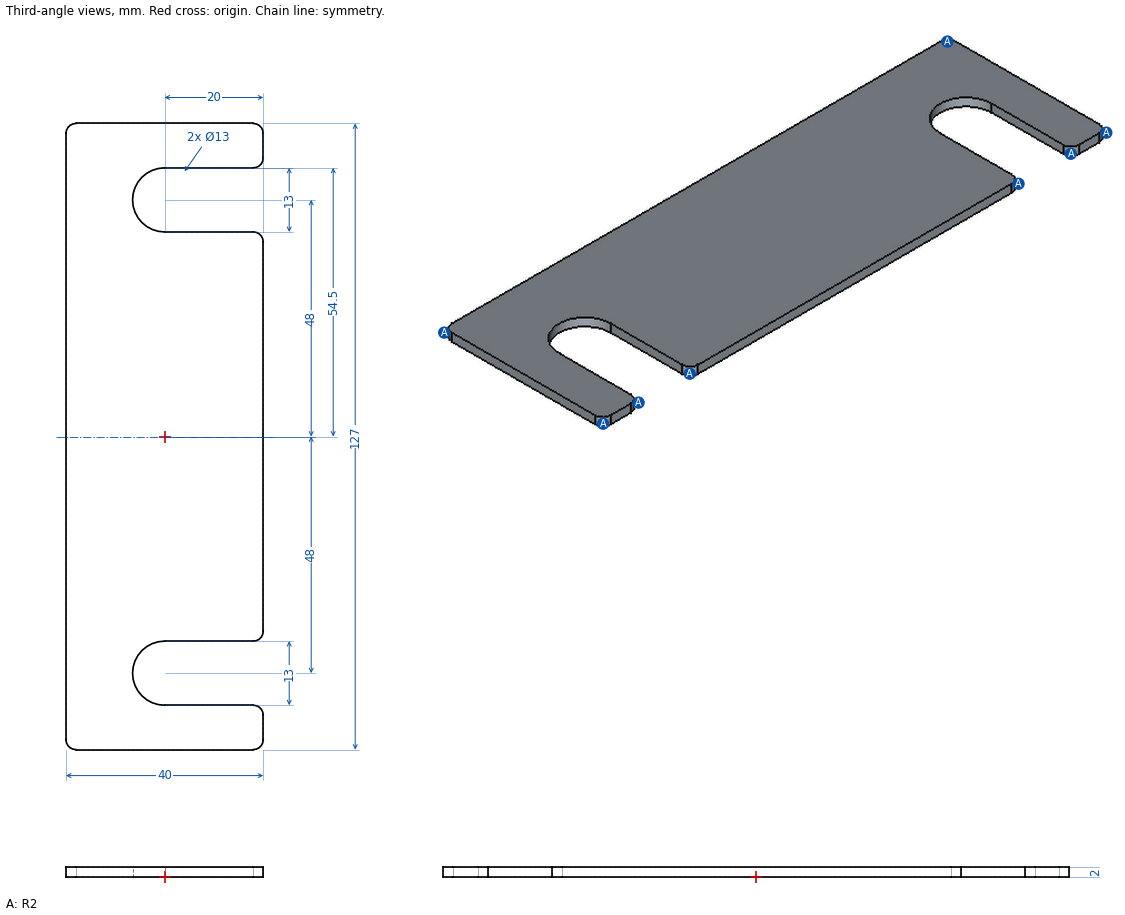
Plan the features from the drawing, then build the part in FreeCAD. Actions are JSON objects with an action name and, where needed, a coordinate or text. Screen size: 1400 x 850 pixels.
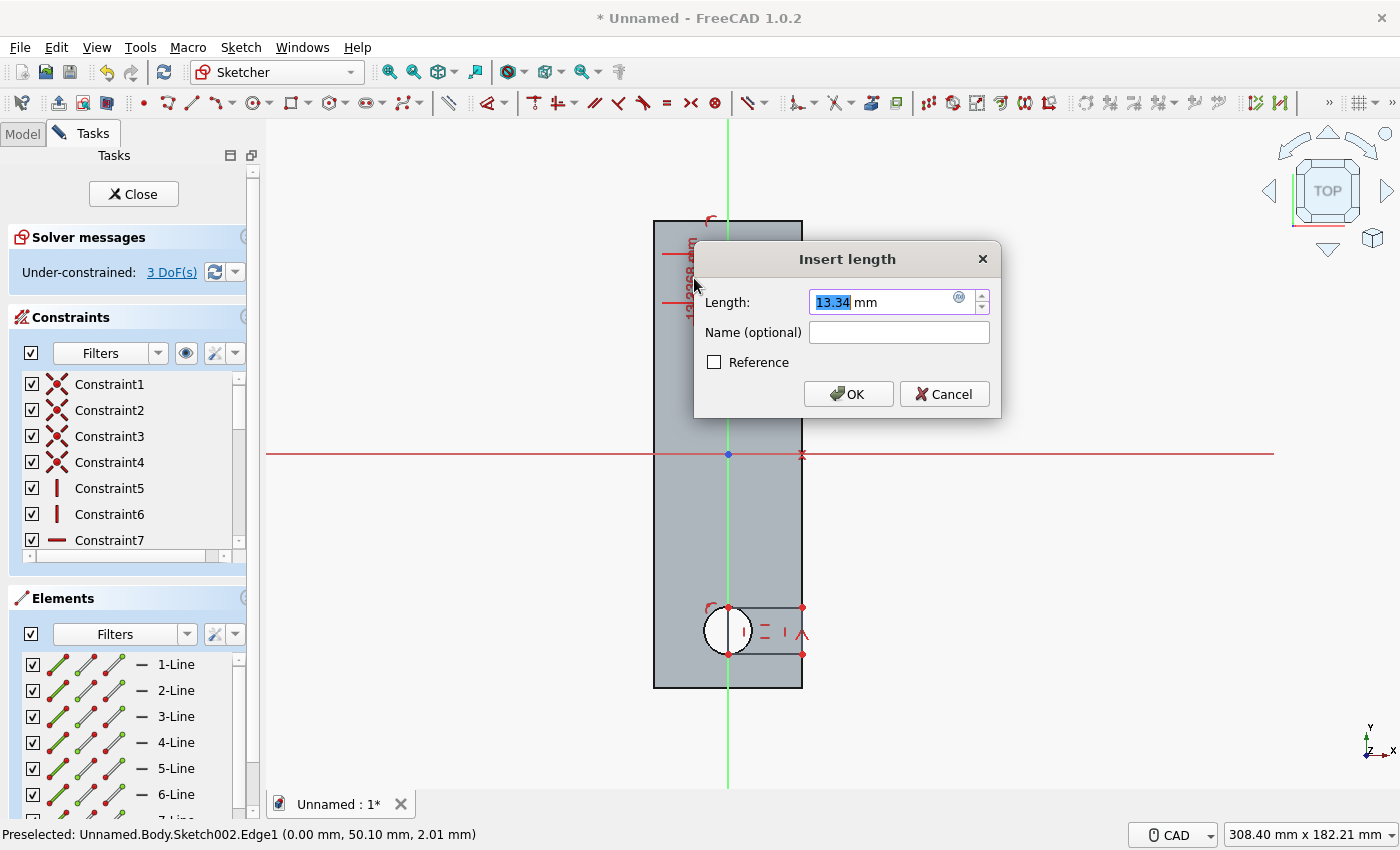
{"action": "type", "text": "13"}
{"action": "key", "text": "Return"}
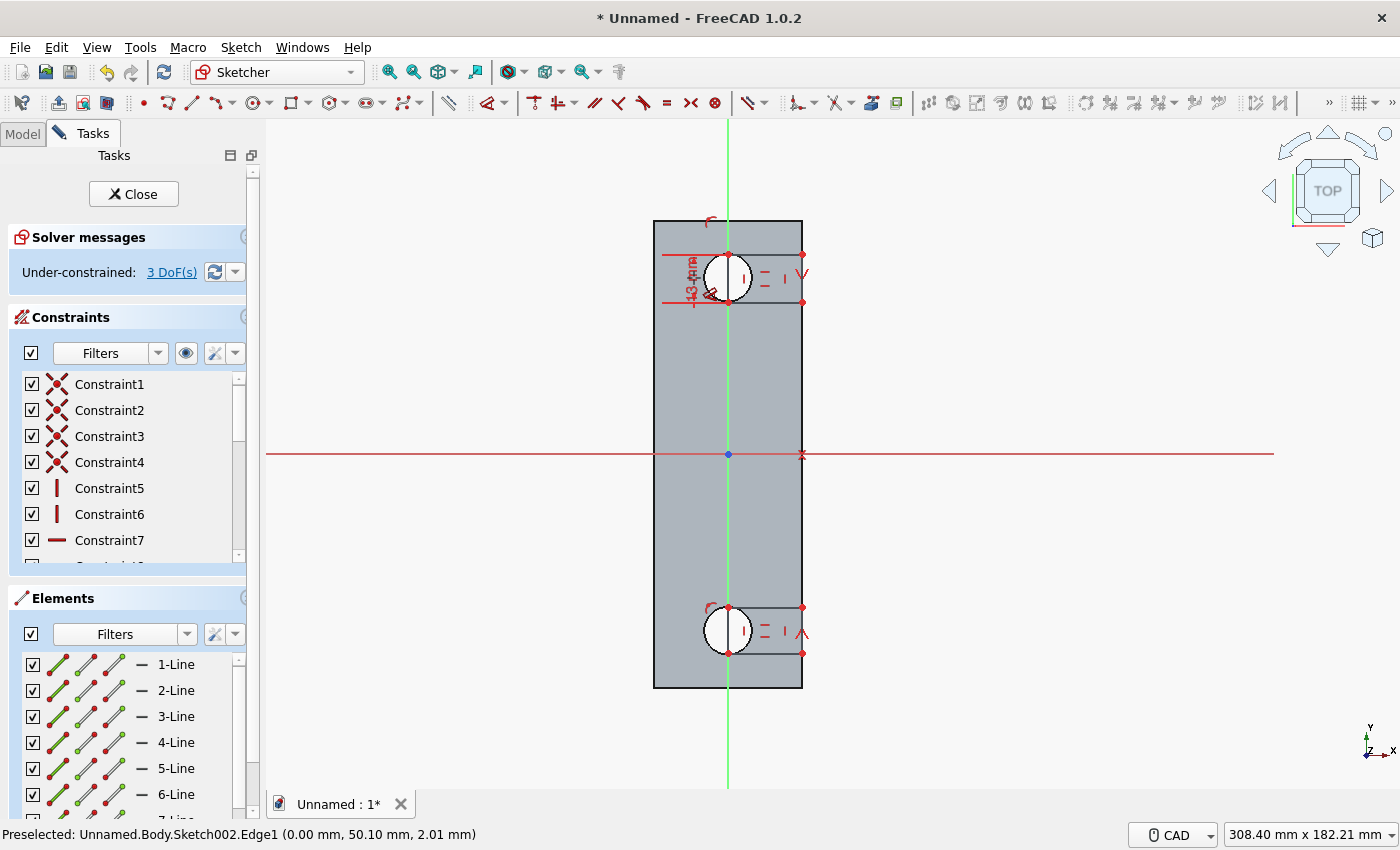
{"action": "left_click", "coordinate": [750, 303]}
{"action": "left_click", "coordinate": [765, 269]}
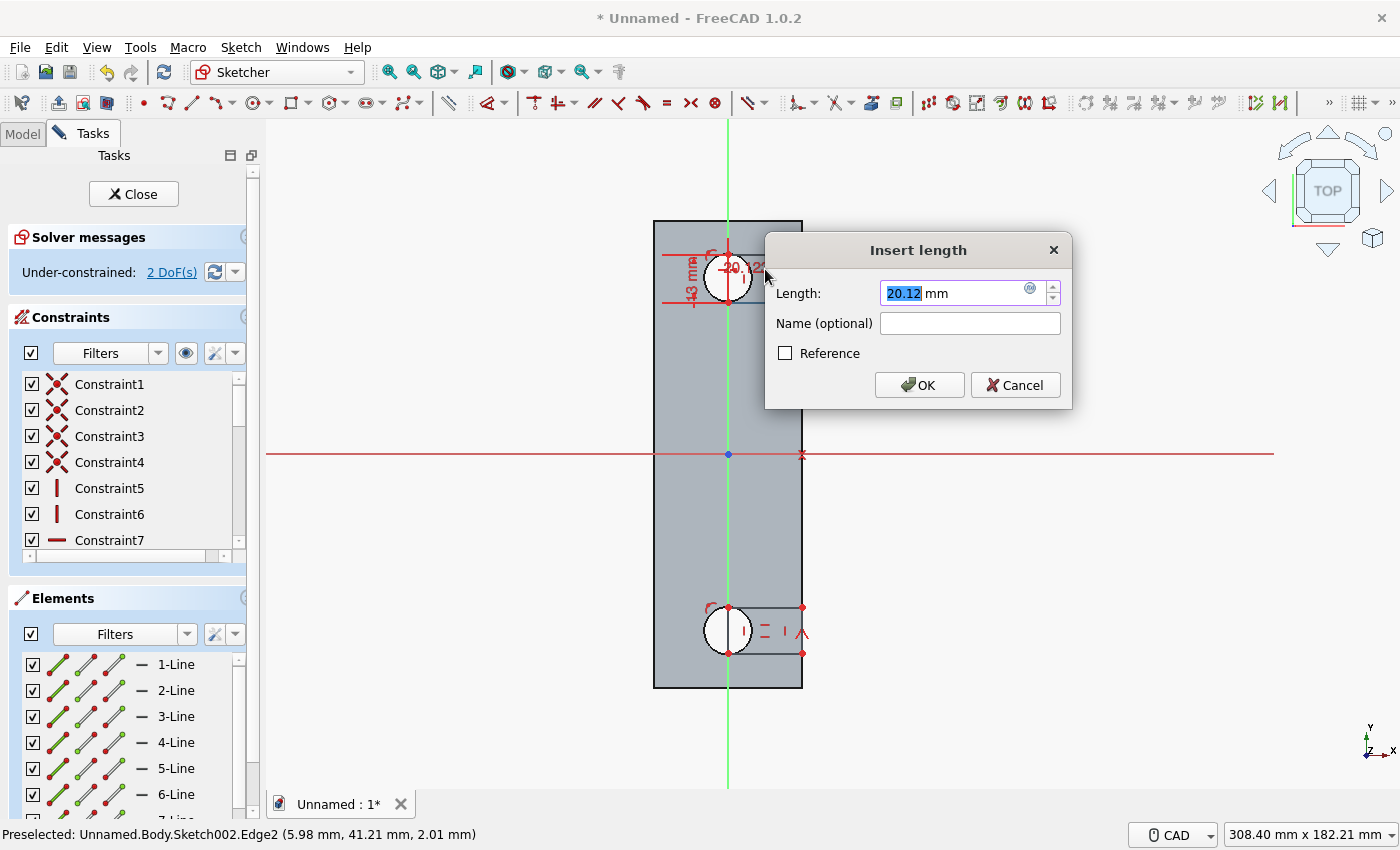
{"action": "type", "text": "20"}
{"action": "key", "text": "Return"}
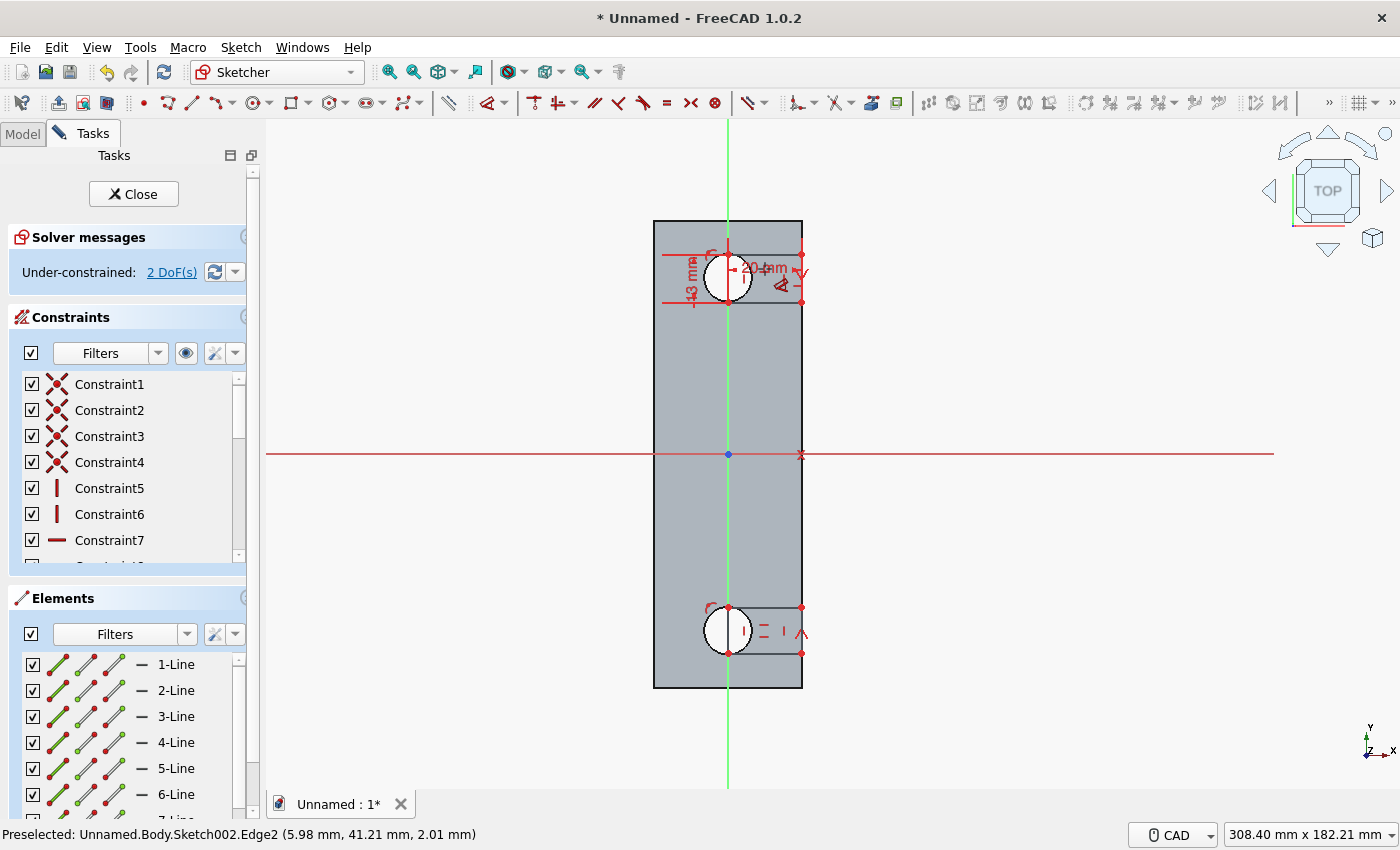
{"action": "left_click", "coordinate": [728, 622]}
{"action": "left_click", "coordinate": [694, 631]}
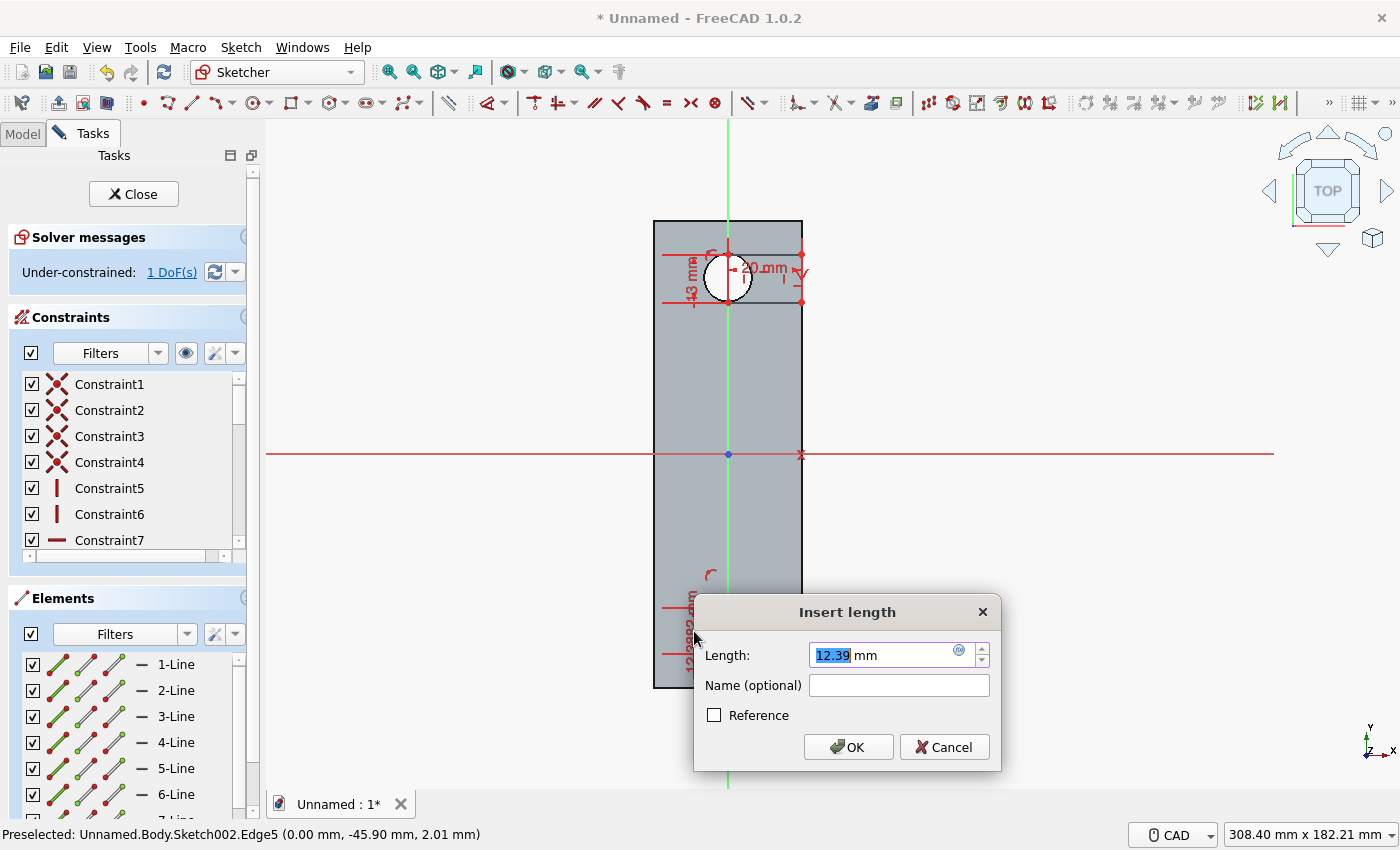
{"action": "type", "text": "13"}
{"action": "key", "text": "Return"}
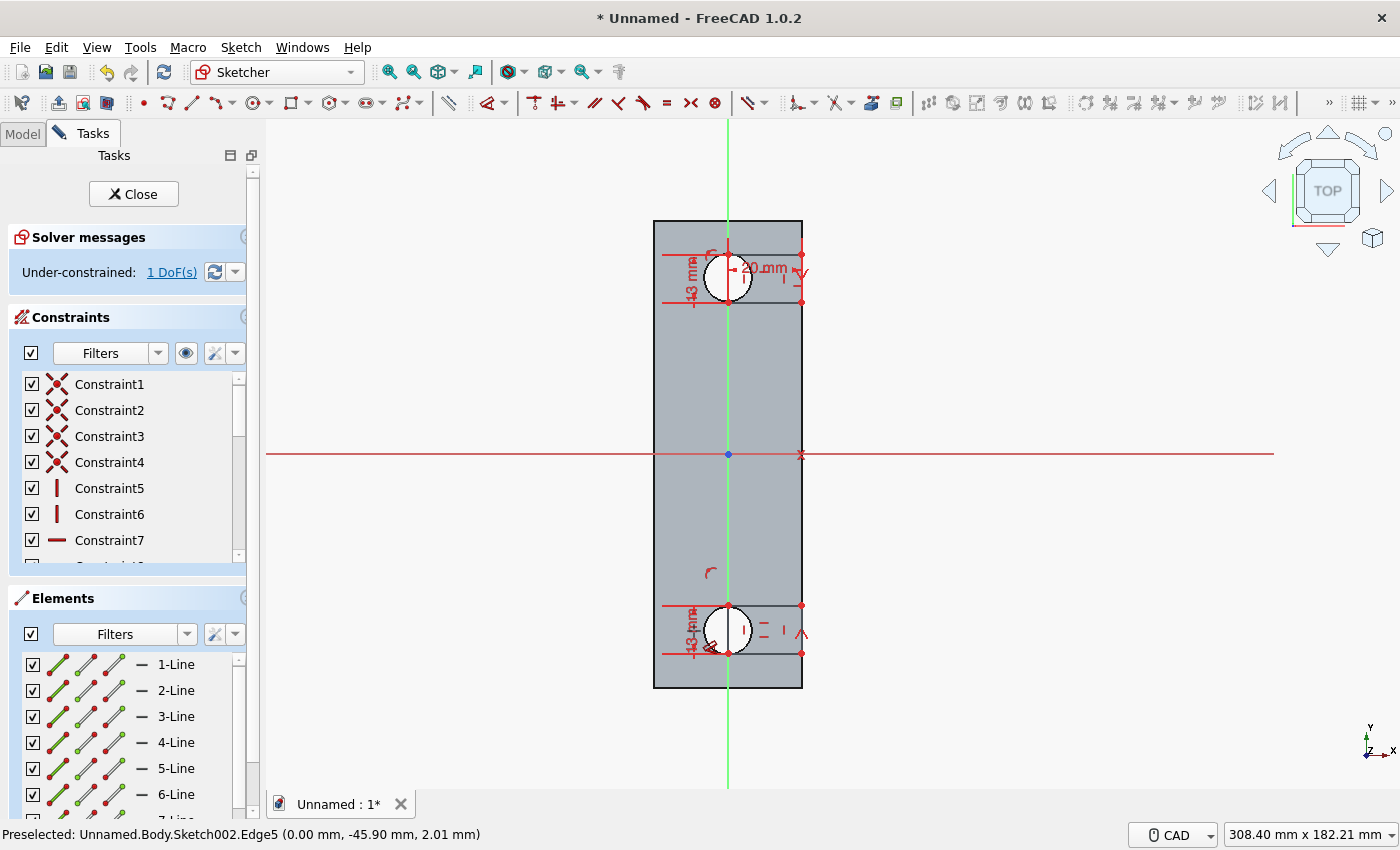
{"action": "left_click", "coordinate": [728, 255]}
{"action": "left_click", "coordinate": [694, 355]}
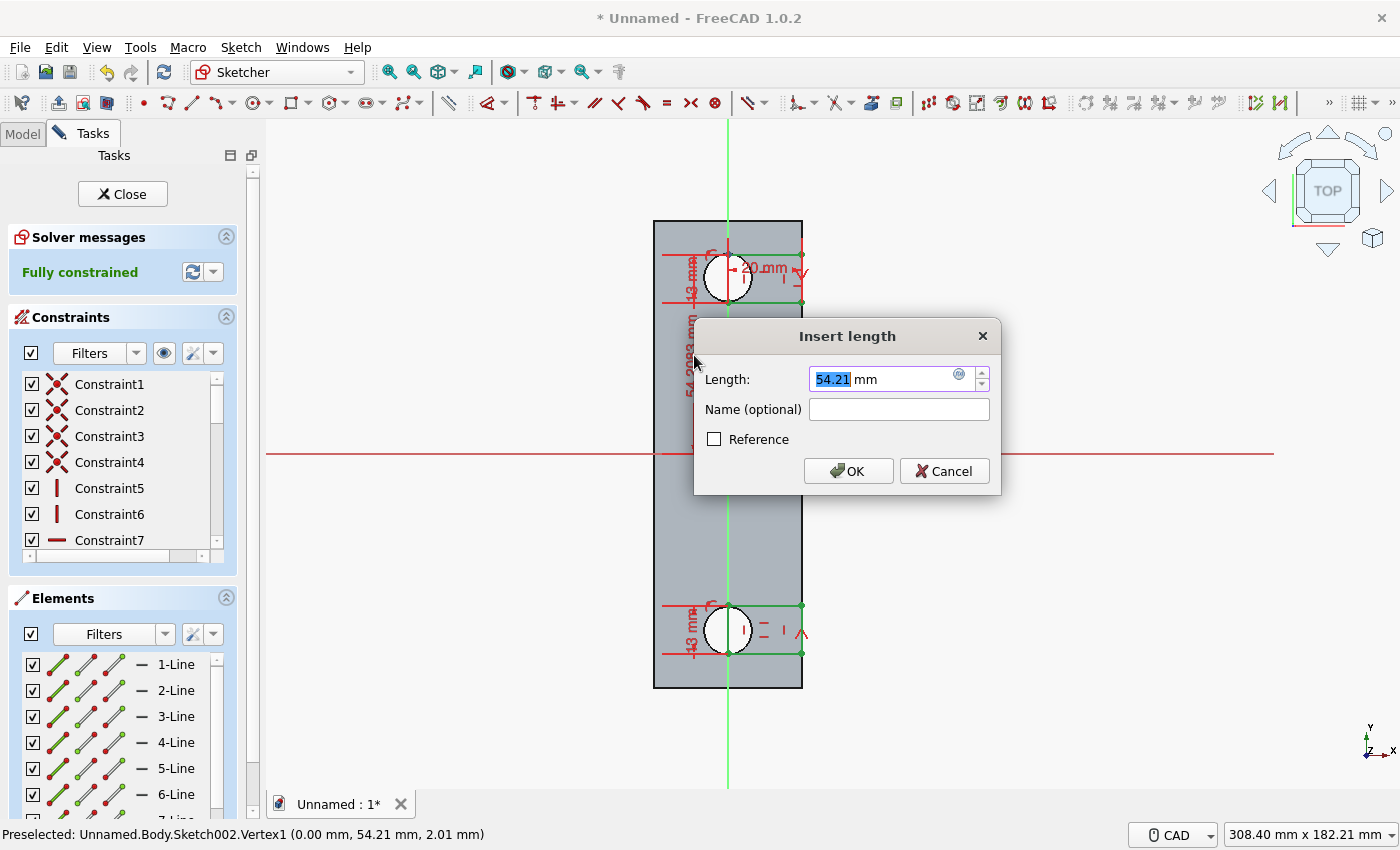
{"action": "type", "text": "54.5"}
{"action": "key", "text": "Return"}
{"action": "key", "text": "Escape"}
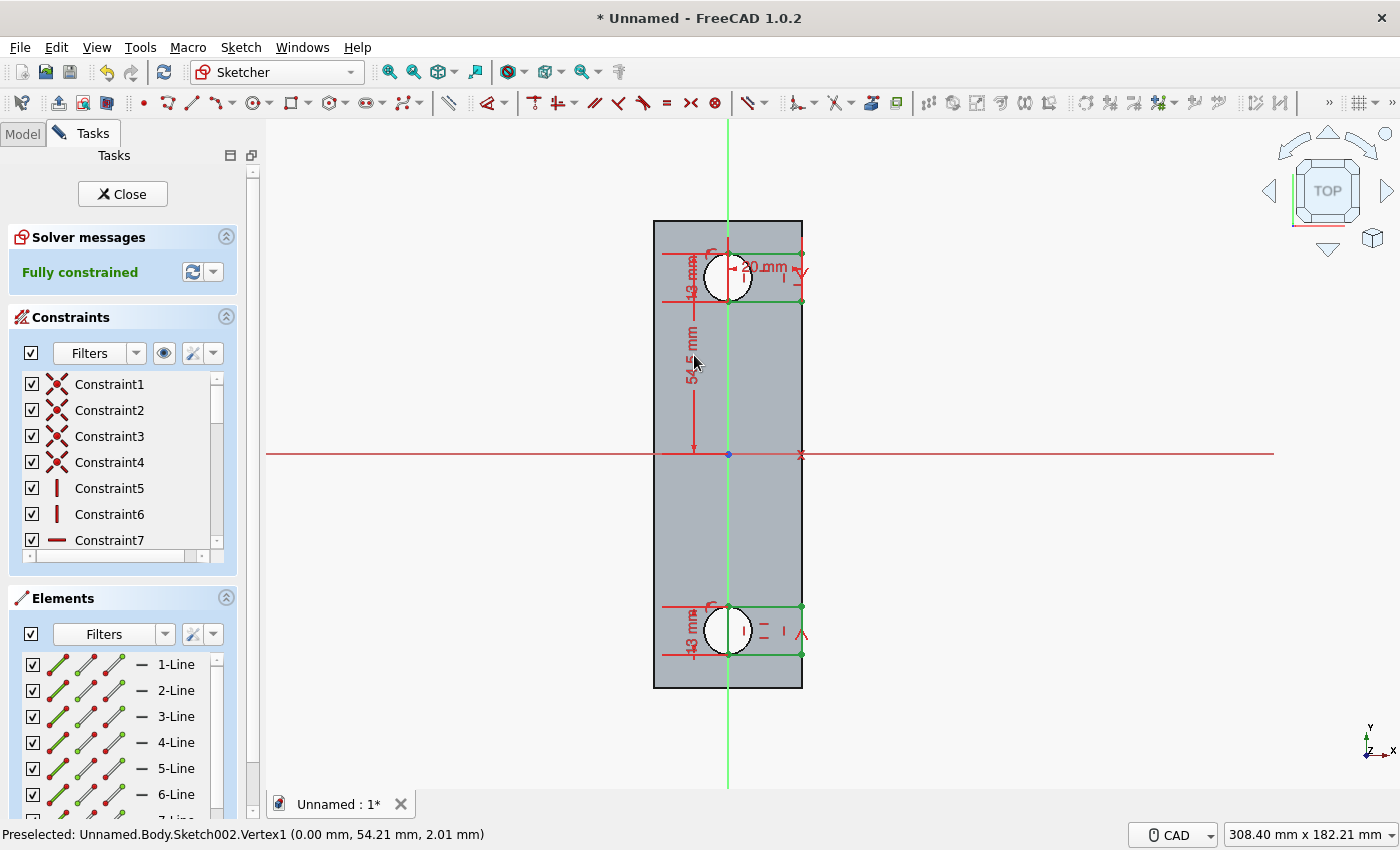
{"action": "left_click", "coordinate": [123, 194]}